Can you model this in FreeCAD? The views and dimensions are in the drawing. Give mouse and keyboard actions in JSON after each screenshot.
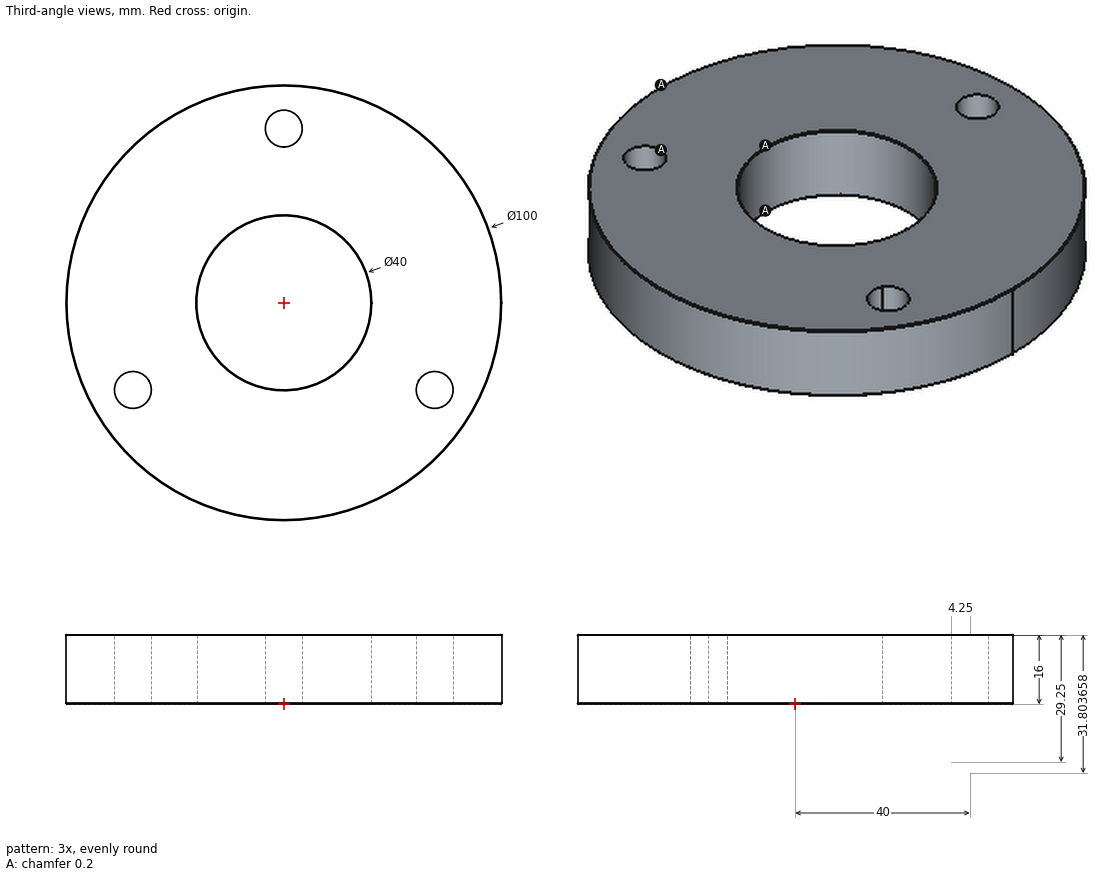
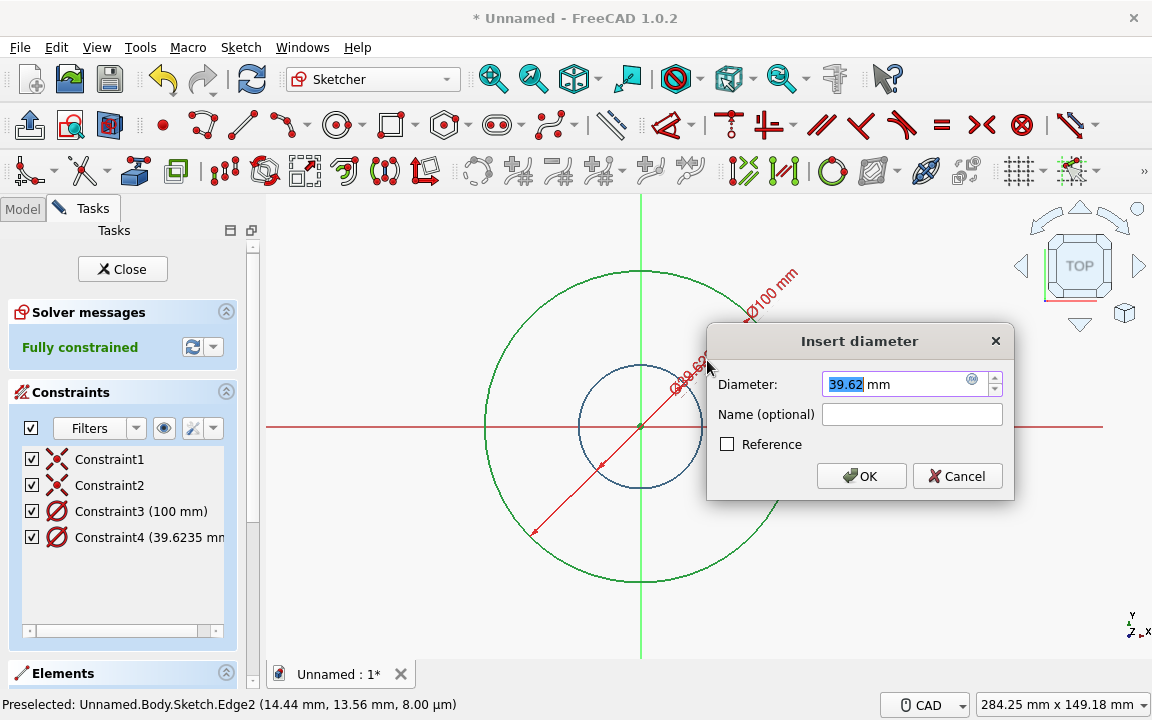
{"action": "type", "text": "40"}
{"action": "key", "text": "Return"}
{"action": "key", "text": "Escape"}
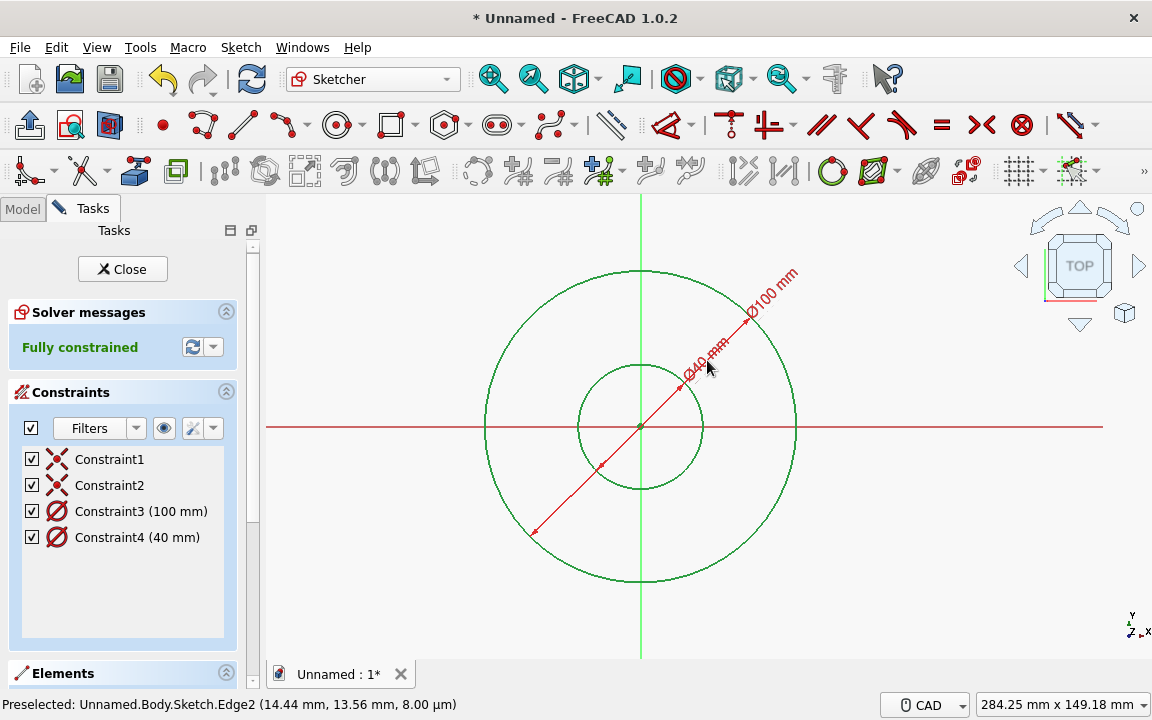
{"action": "left_click", "coordinate": [123, 269]}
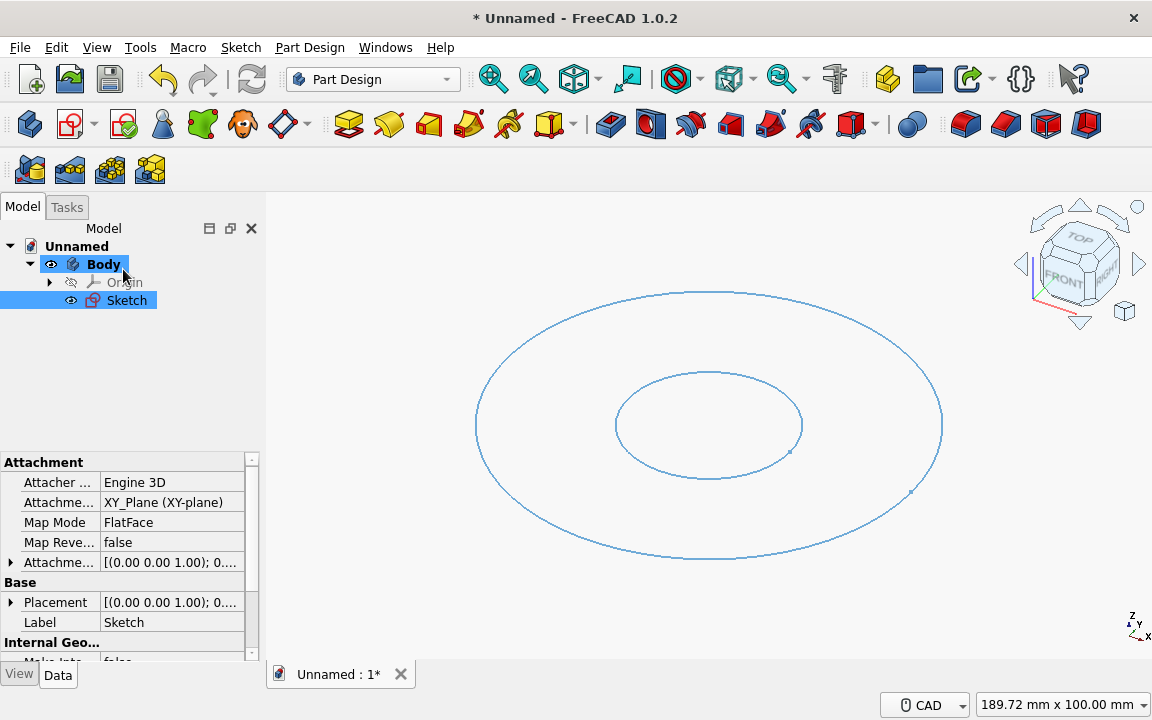
{"action": "left_click", "coordinate": [350, 124]}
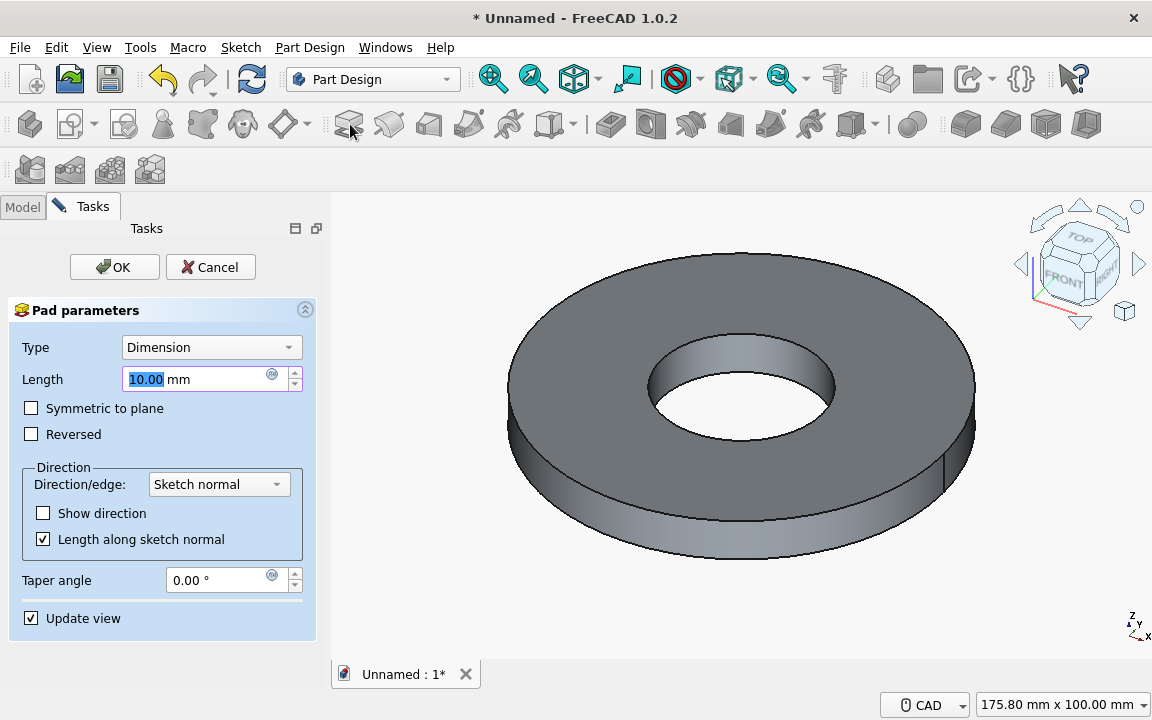
{"action": "type", "text": "16"}
{"action": "key", "text": "Tab"}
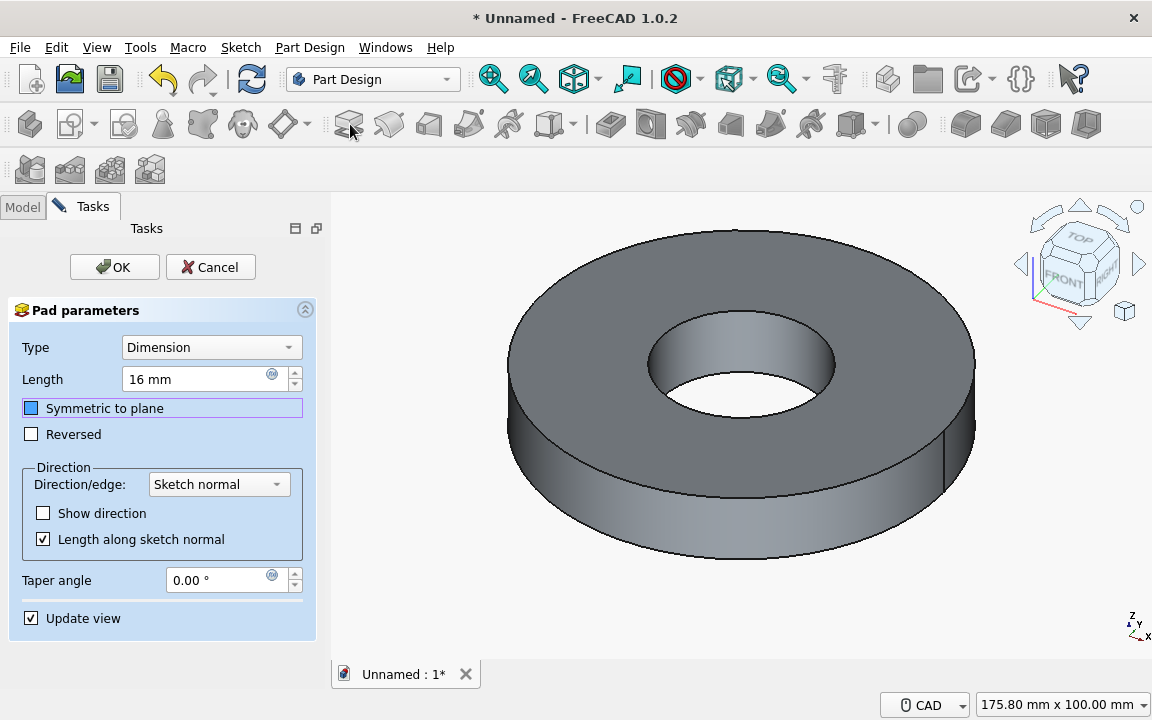
{"action": "left_click", "coordinate": [115, 267]}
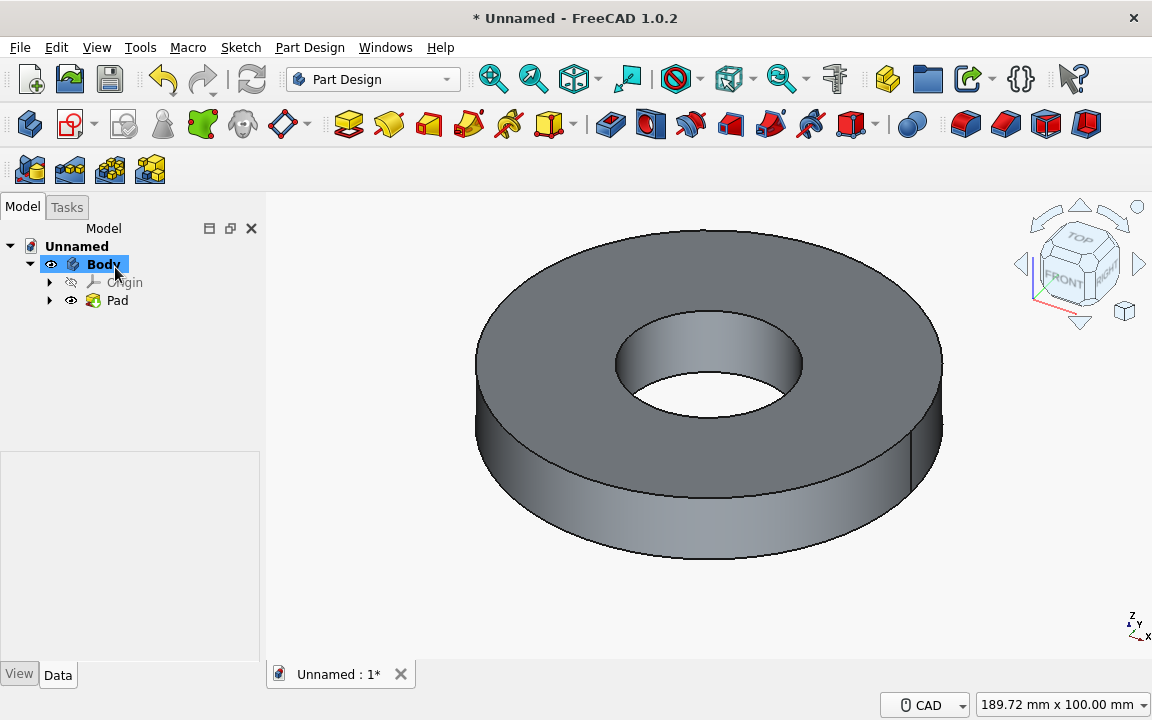
{"action": "left_click", "coordinate": [494, 80]}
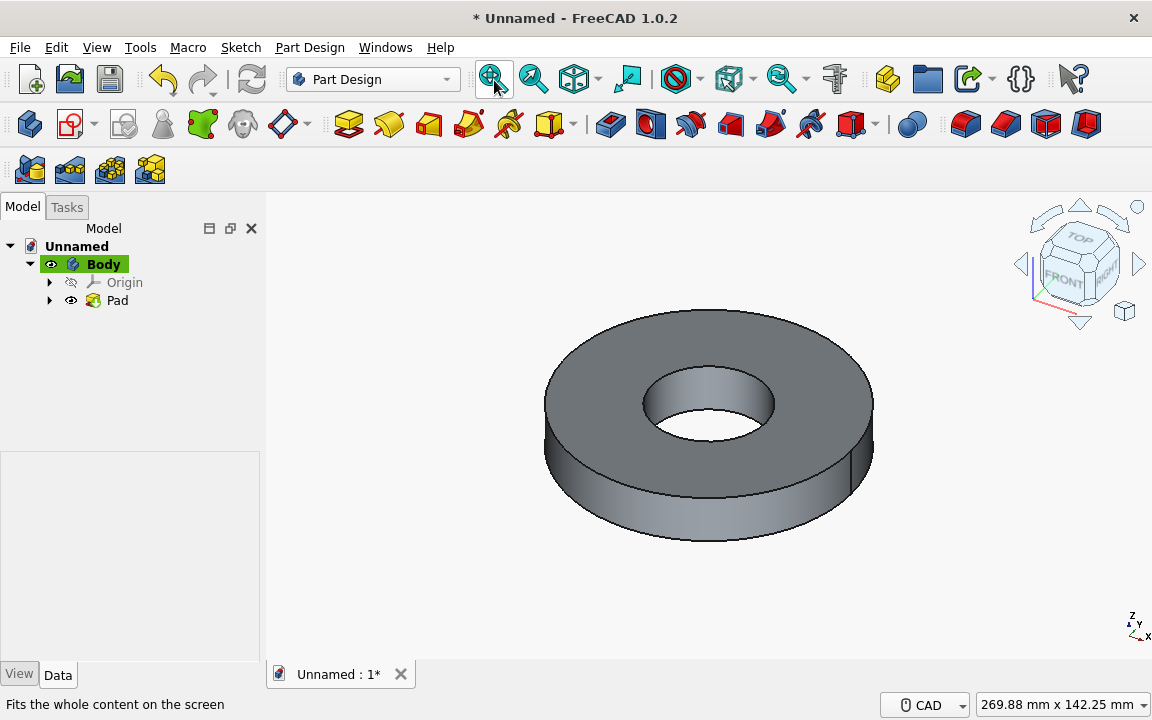
{"action": "left_click", "coordinate": [70, 124]}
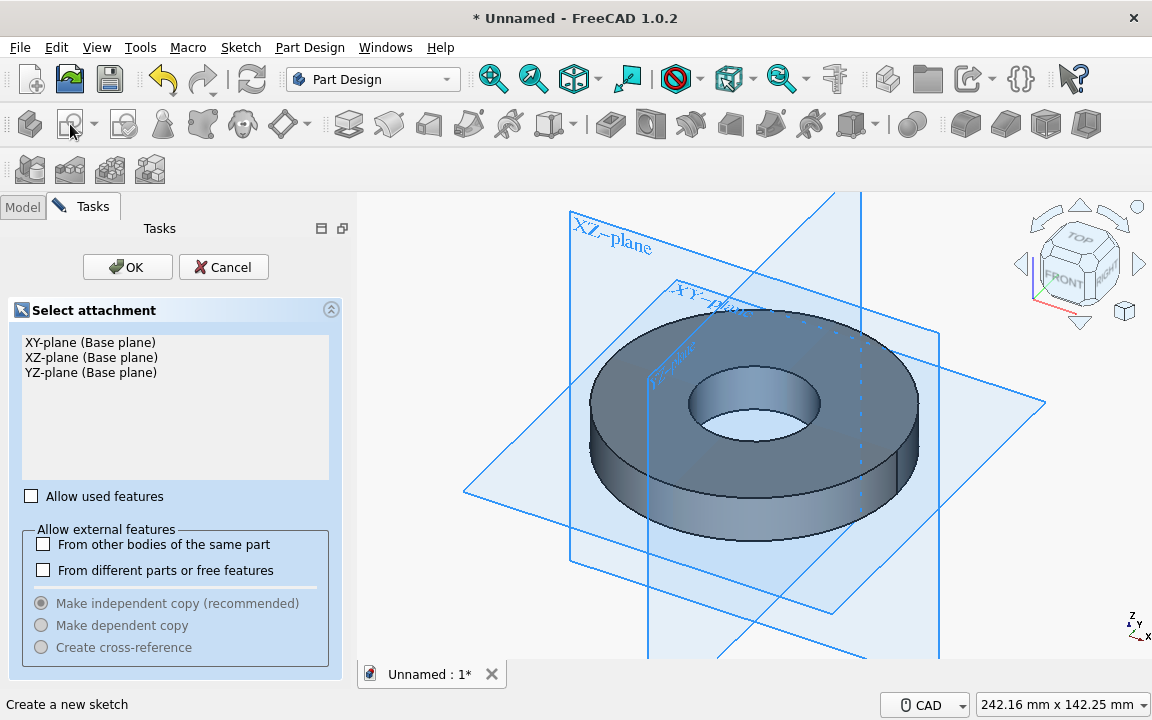
{"action": "left_click", "coordinate": [82, 372]}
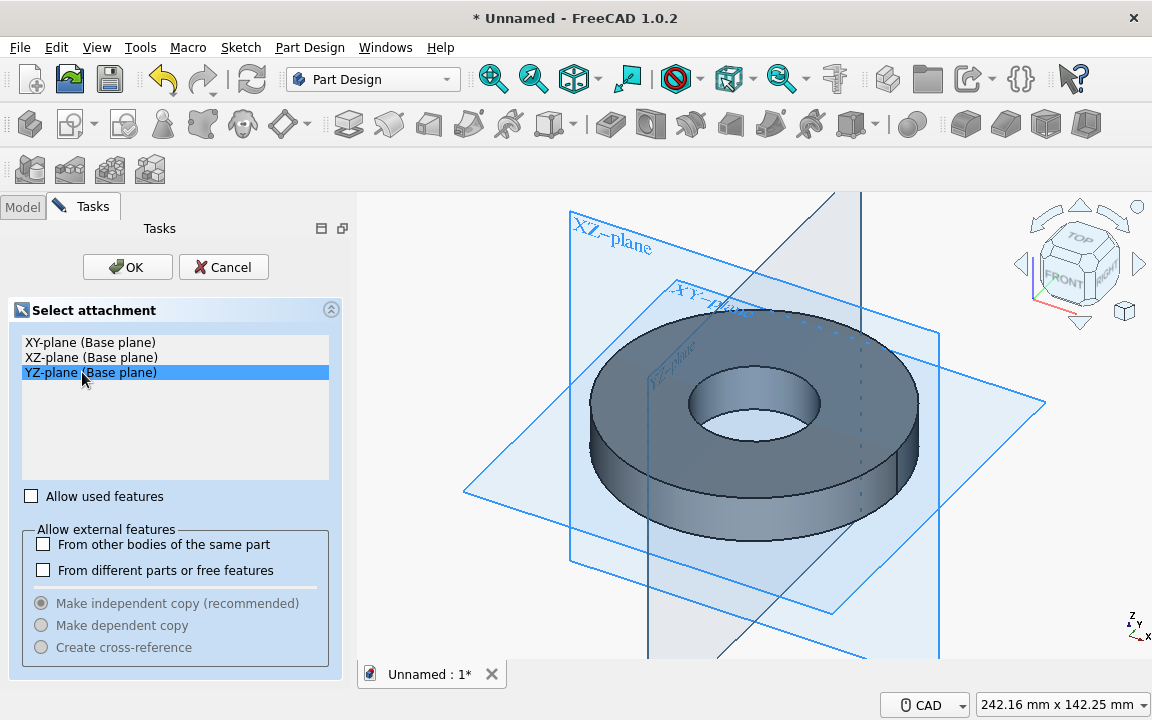
{"action": "left_click", "coordinate": [128, 267]}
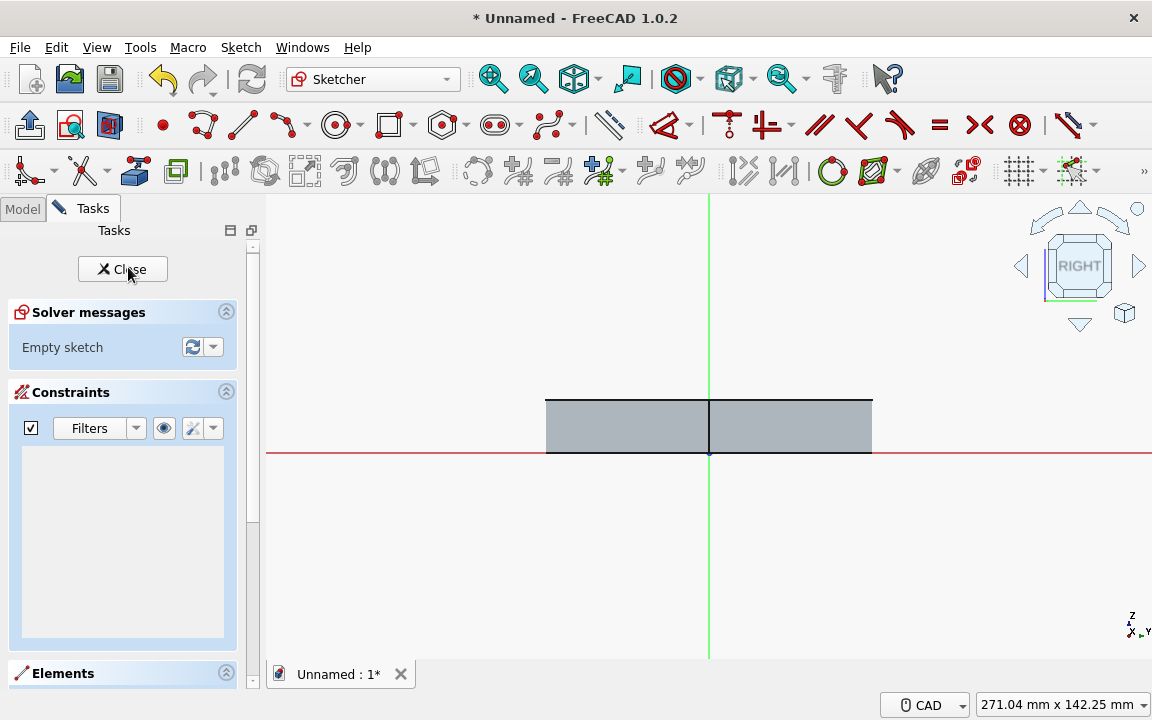
{"action": "left_click", "coordinate": [110, 126]}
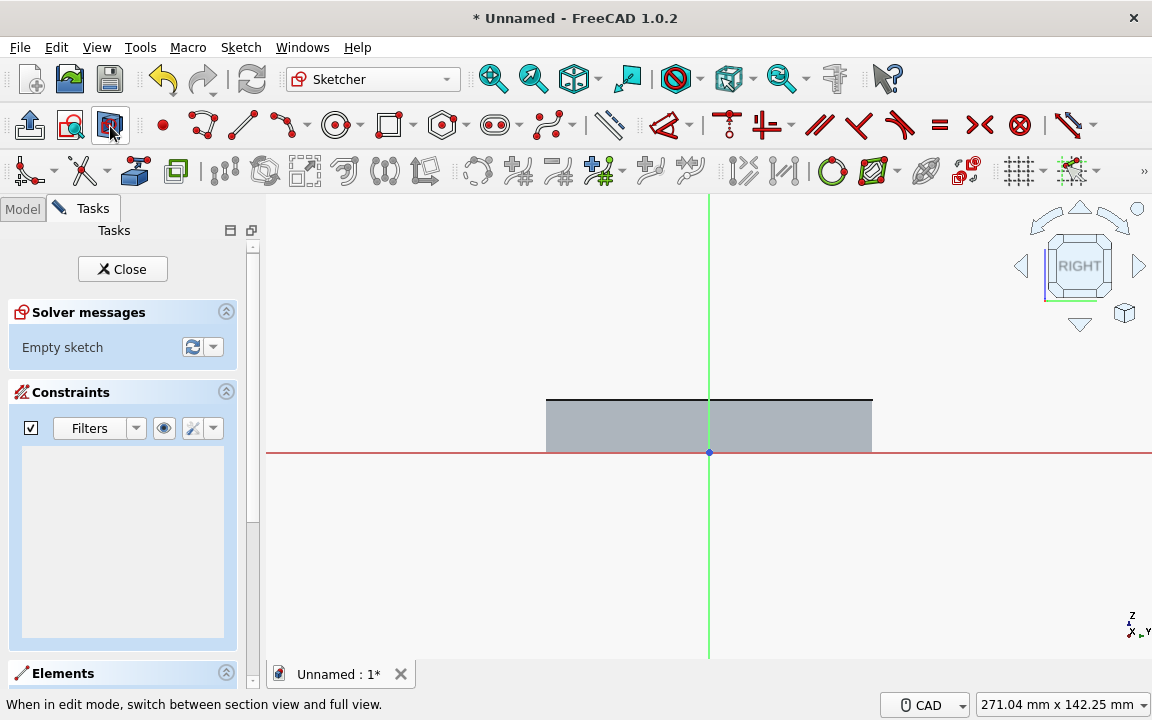
{"action": "scroll", "coordinate": [937, 530], "scroll_direction": "up", "scroll_amount": 3}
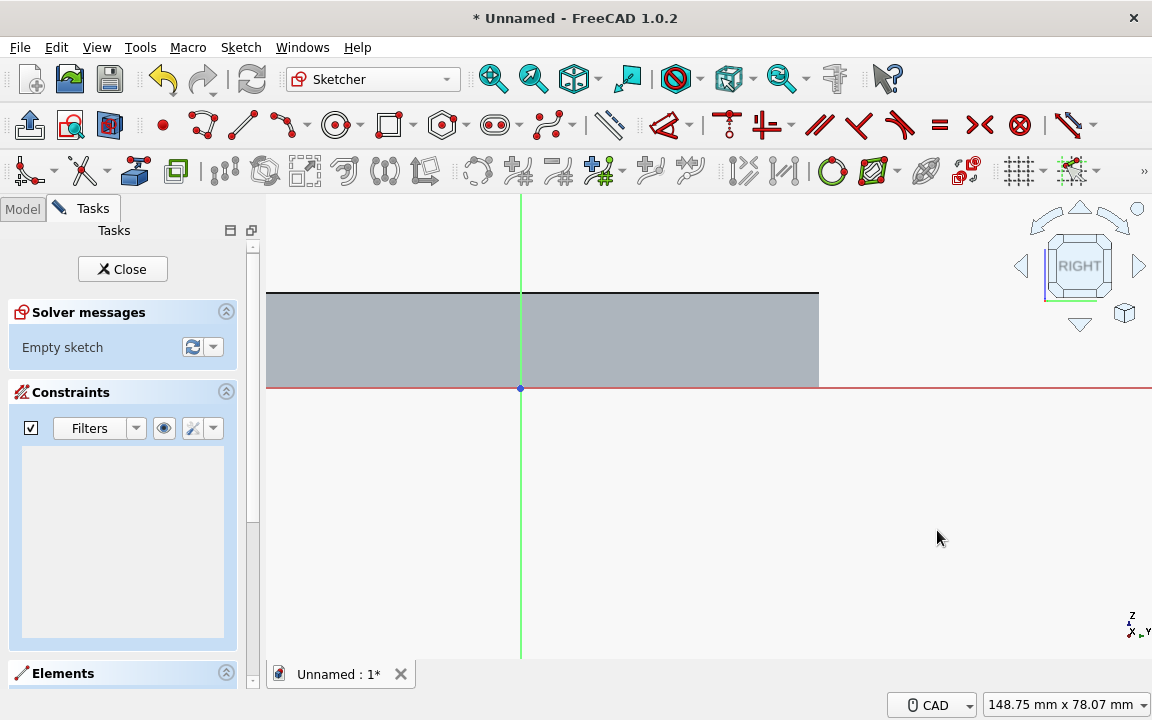
{"action": "left_click", "coordinate": [204, 126]}